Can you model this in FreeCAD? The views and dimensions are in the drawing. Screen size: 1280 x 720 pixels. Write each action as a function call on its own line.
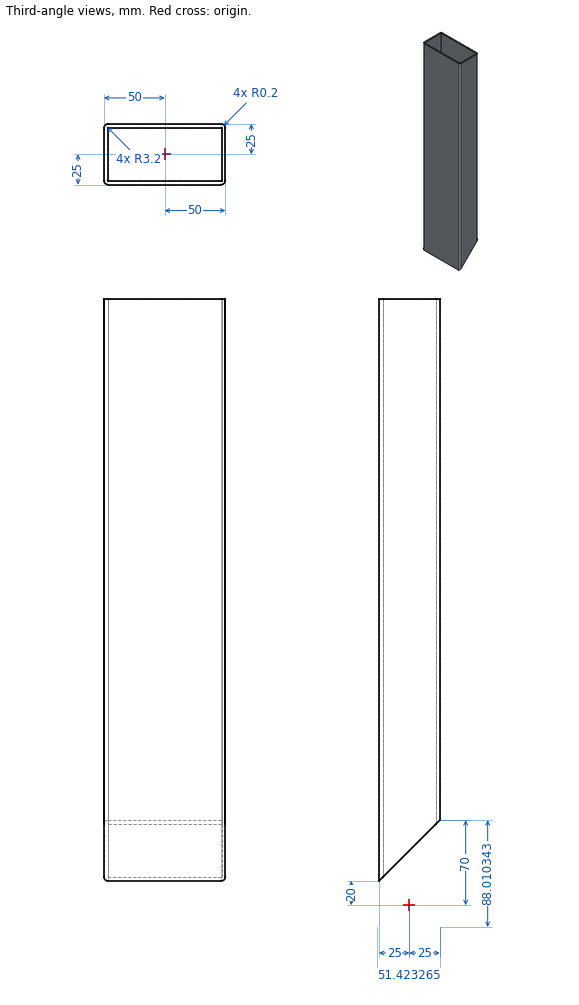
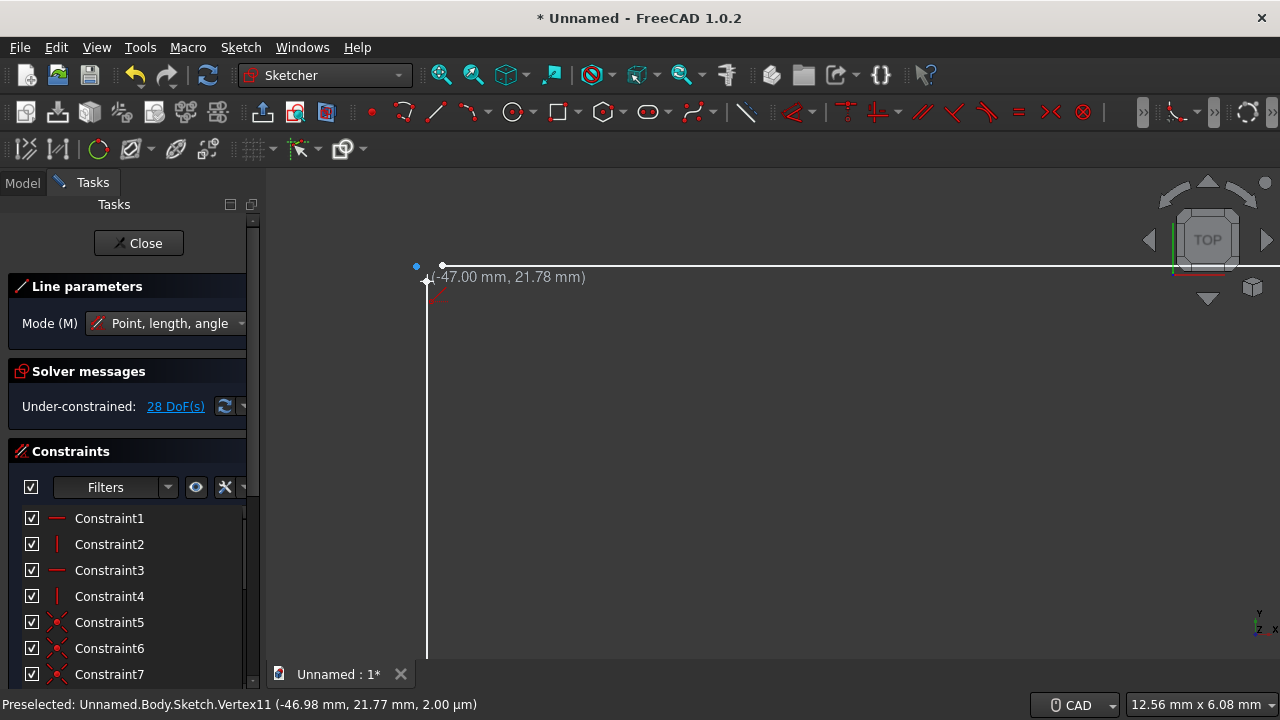
click(468, 112)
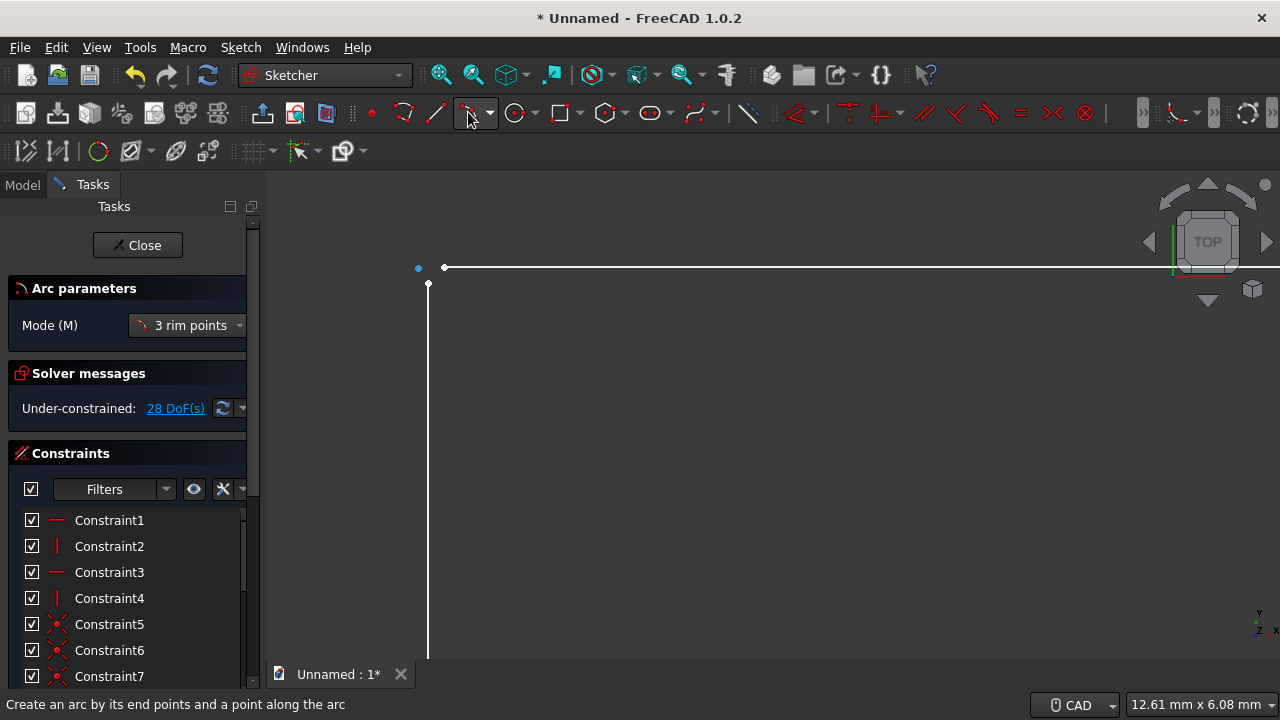
scroll(423, 284, down, 13)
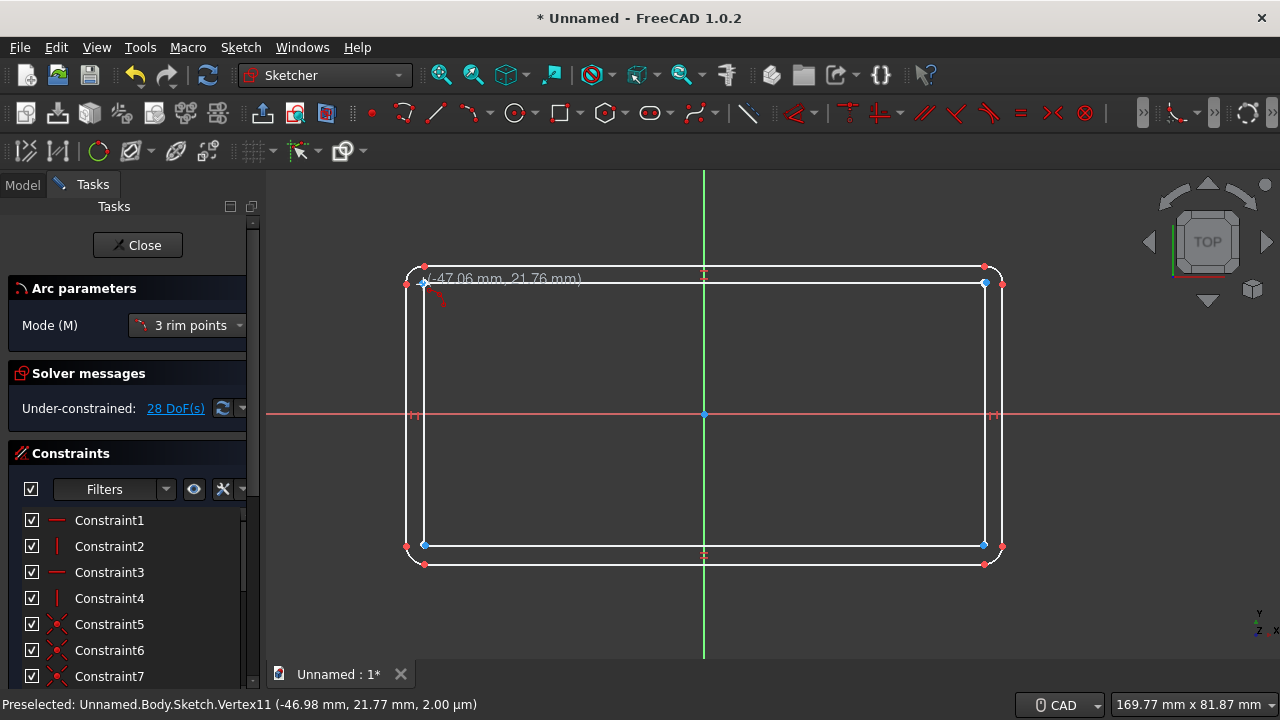
scroll(984, 283, up, 13)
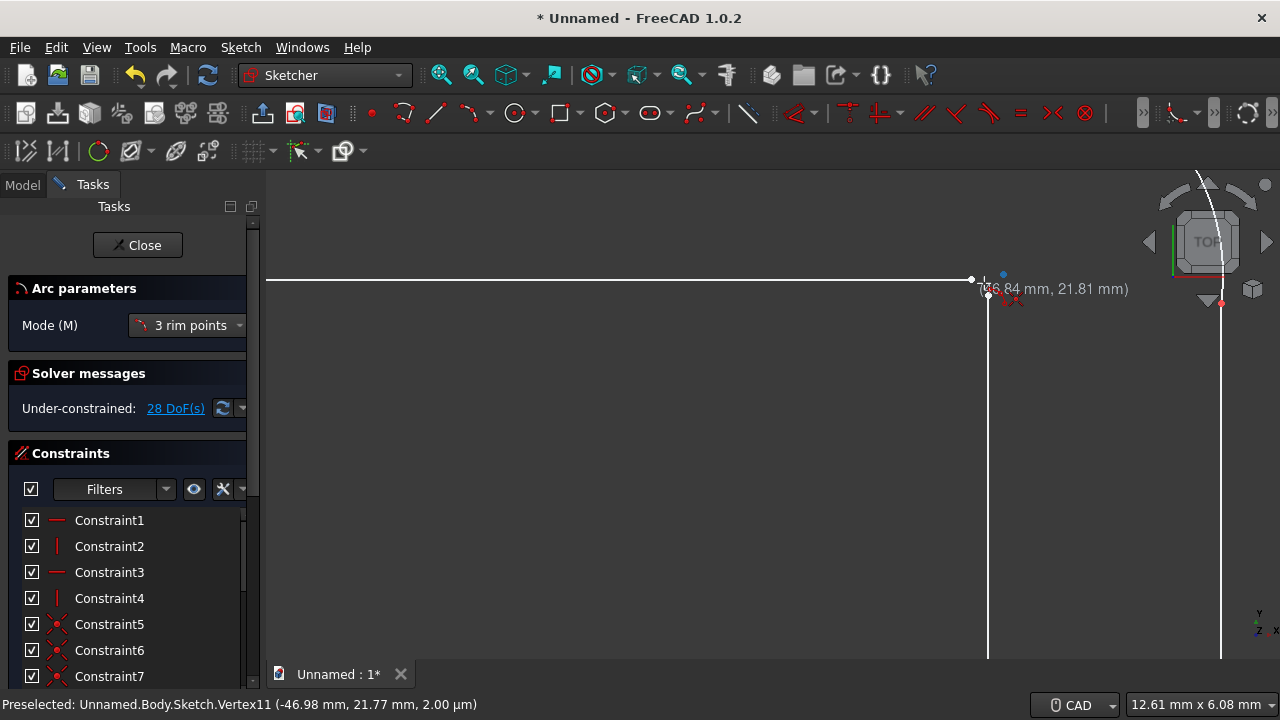
click(972, 280)
click(988, 296)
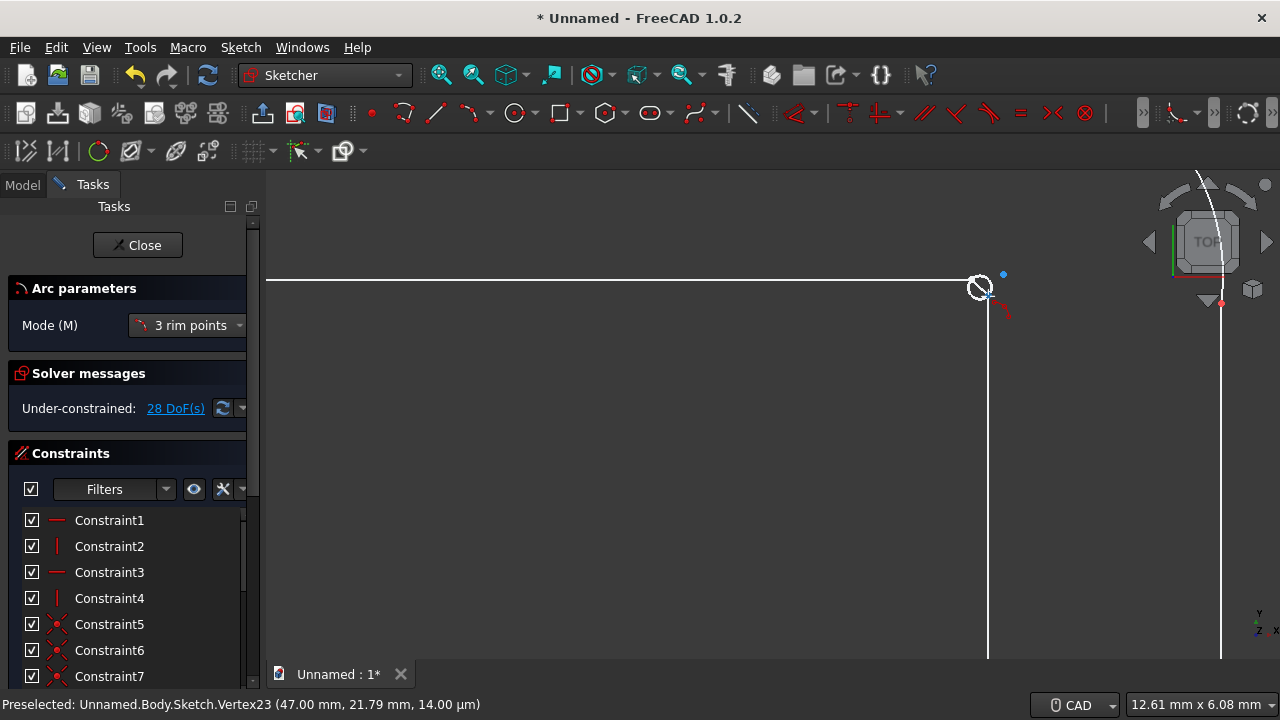
scroll(983, 283, up, 7)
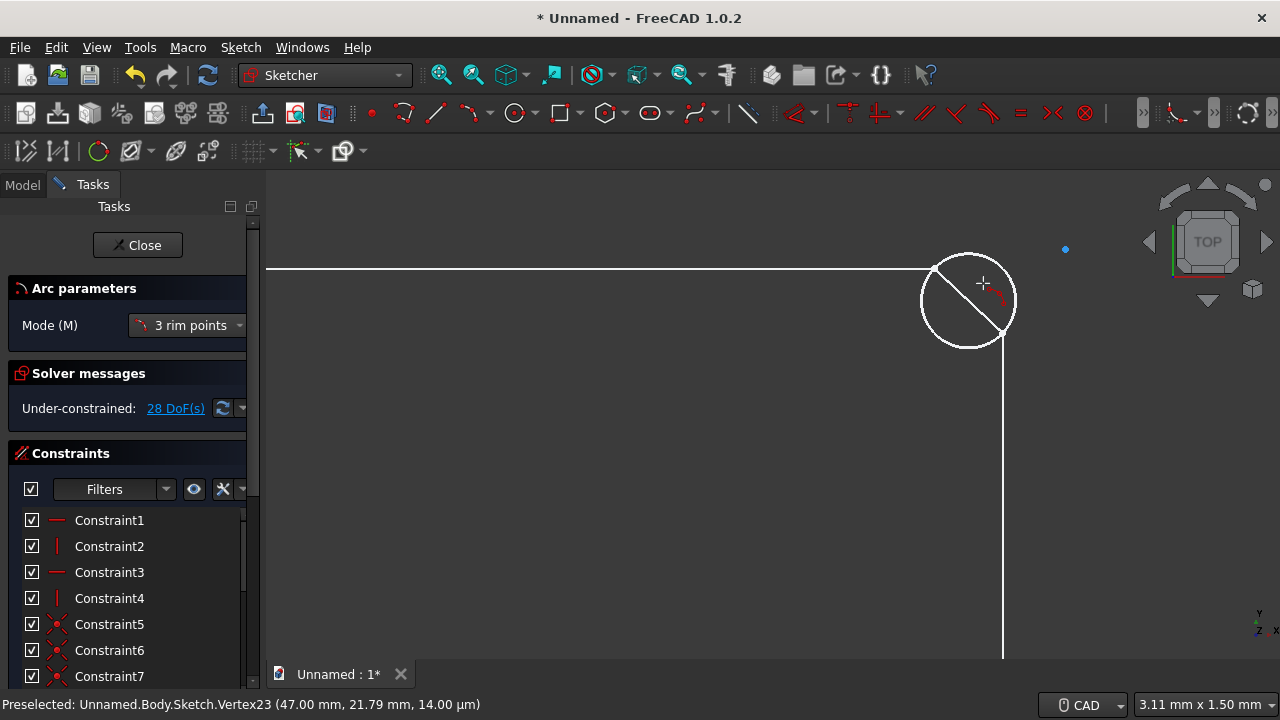
click(982, 283)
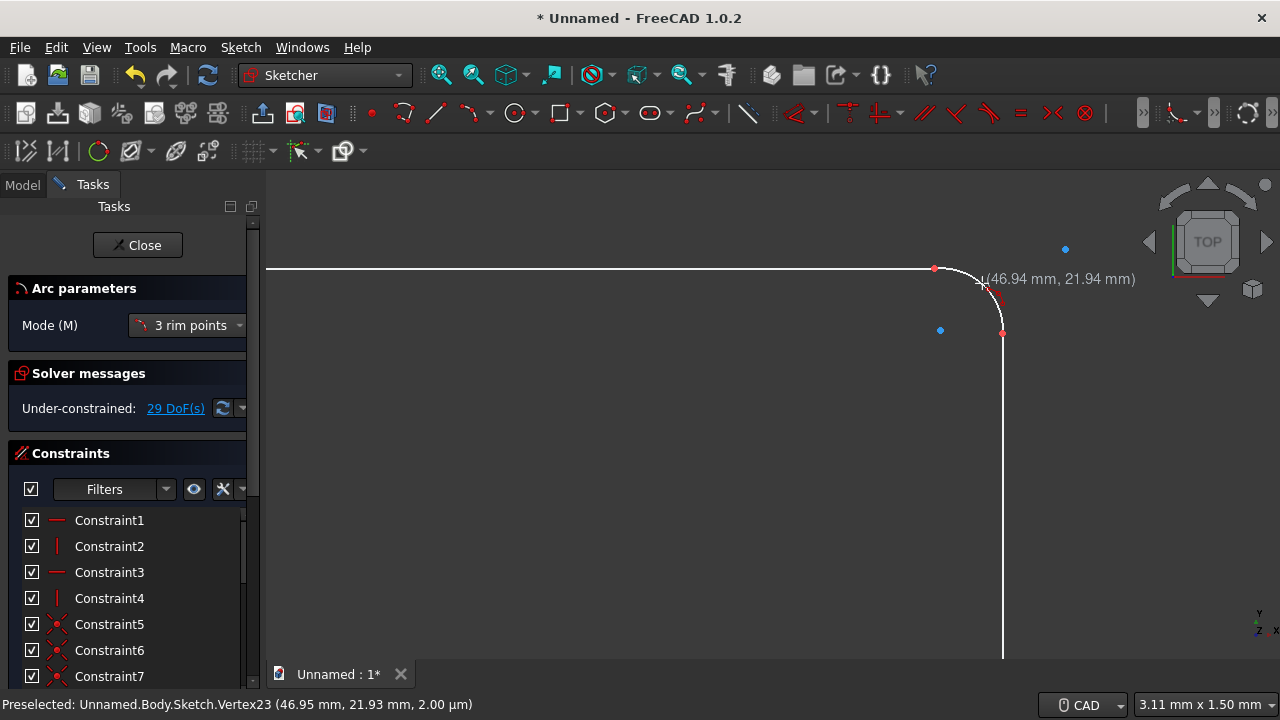
scroll(704, 414, down, 15)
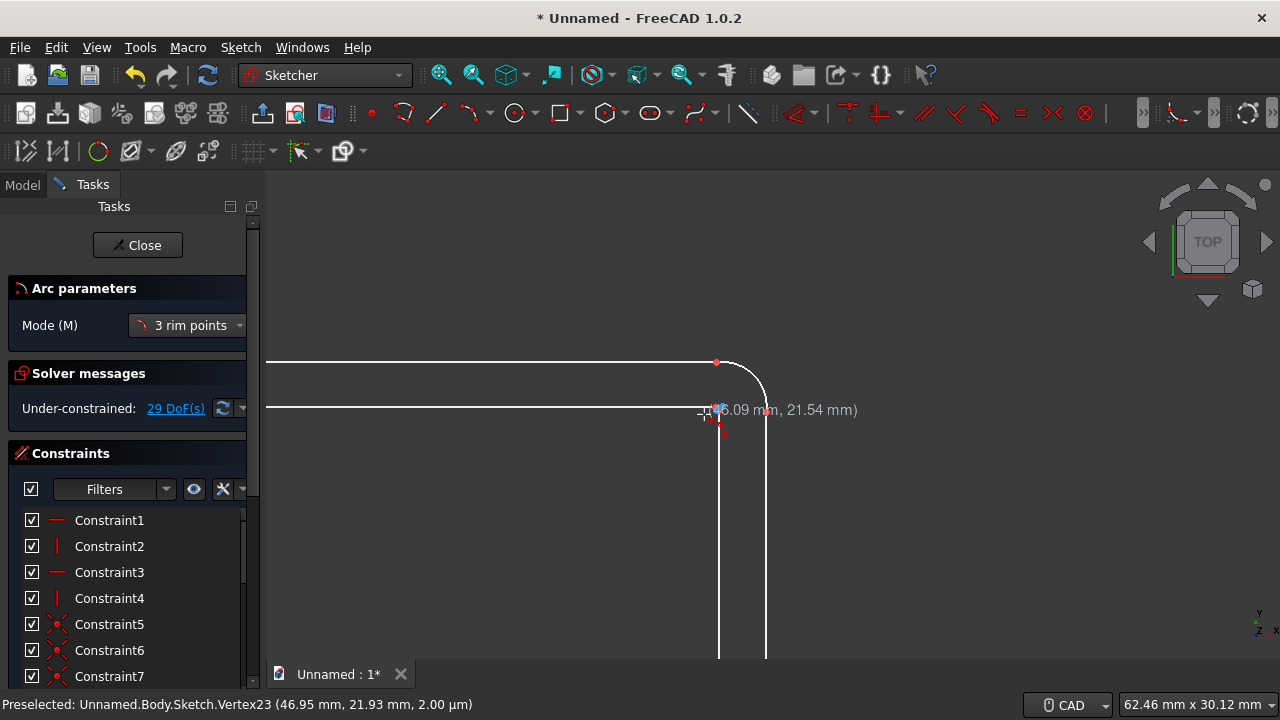
scroll(1115, 211, down, 5)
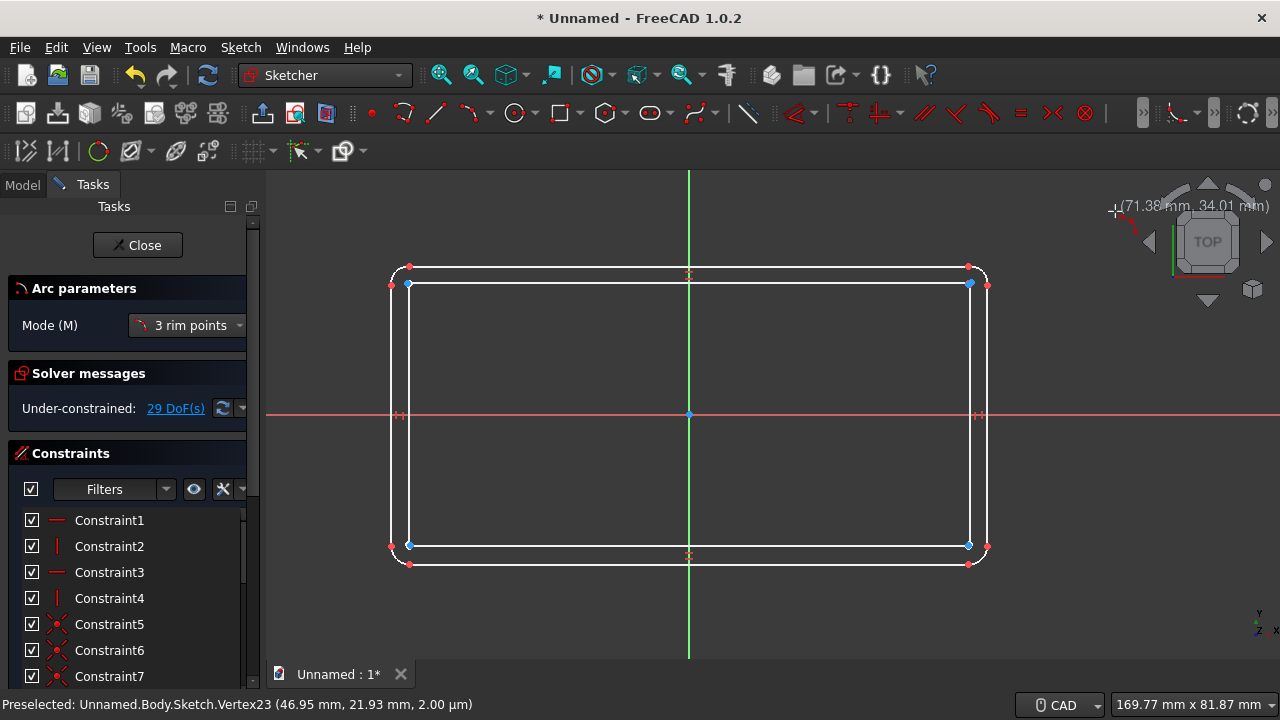
scroll(970, 545, up, 13)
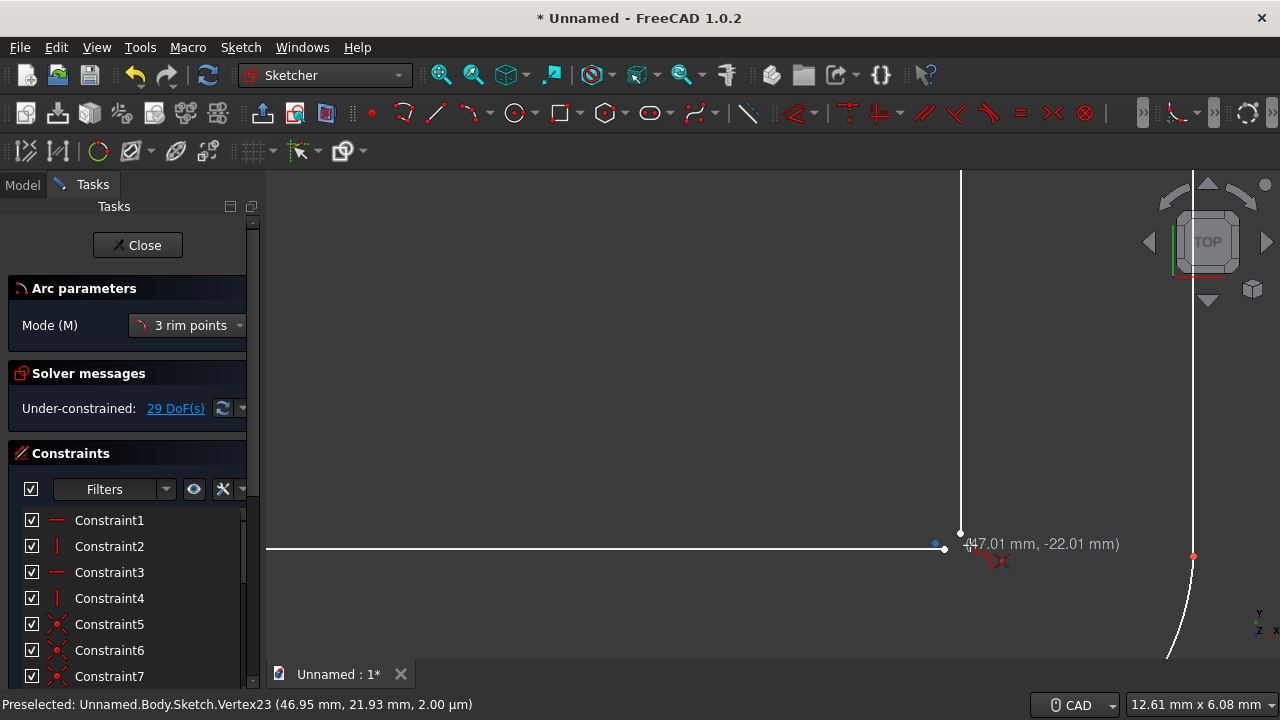
click(961, 533)
click(944, 549)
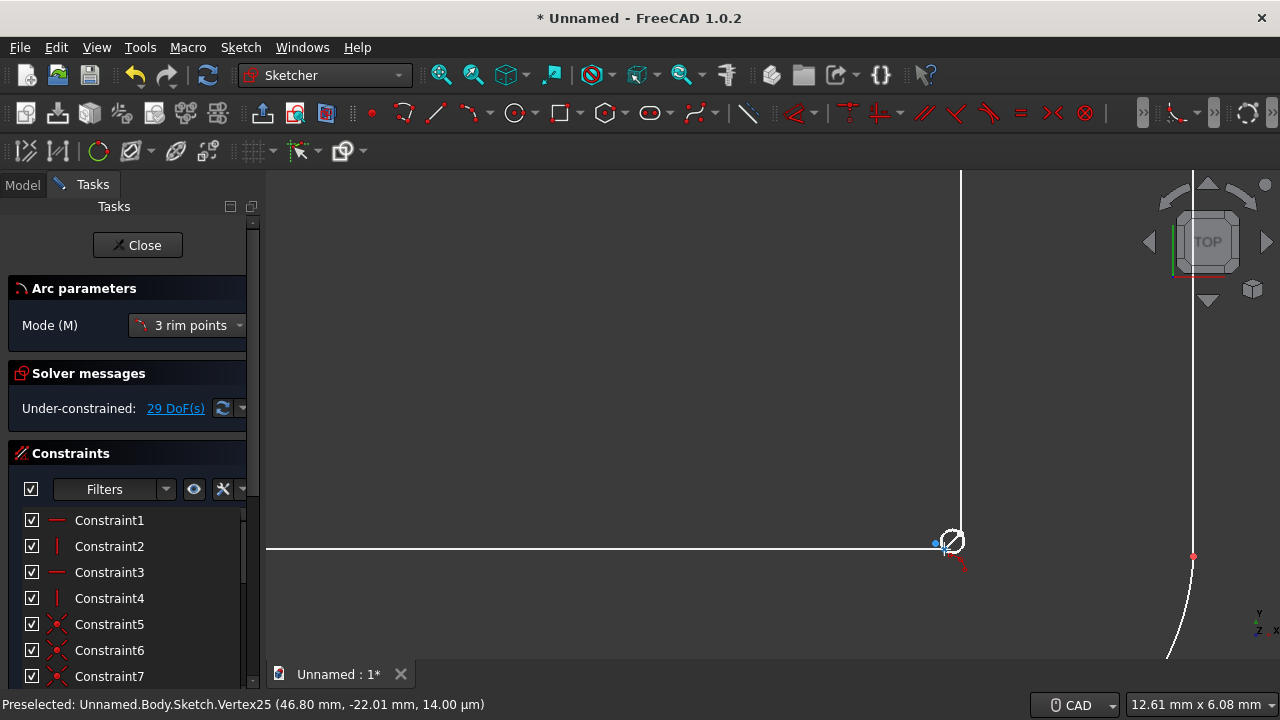
scroll(956, 544, up, 7)